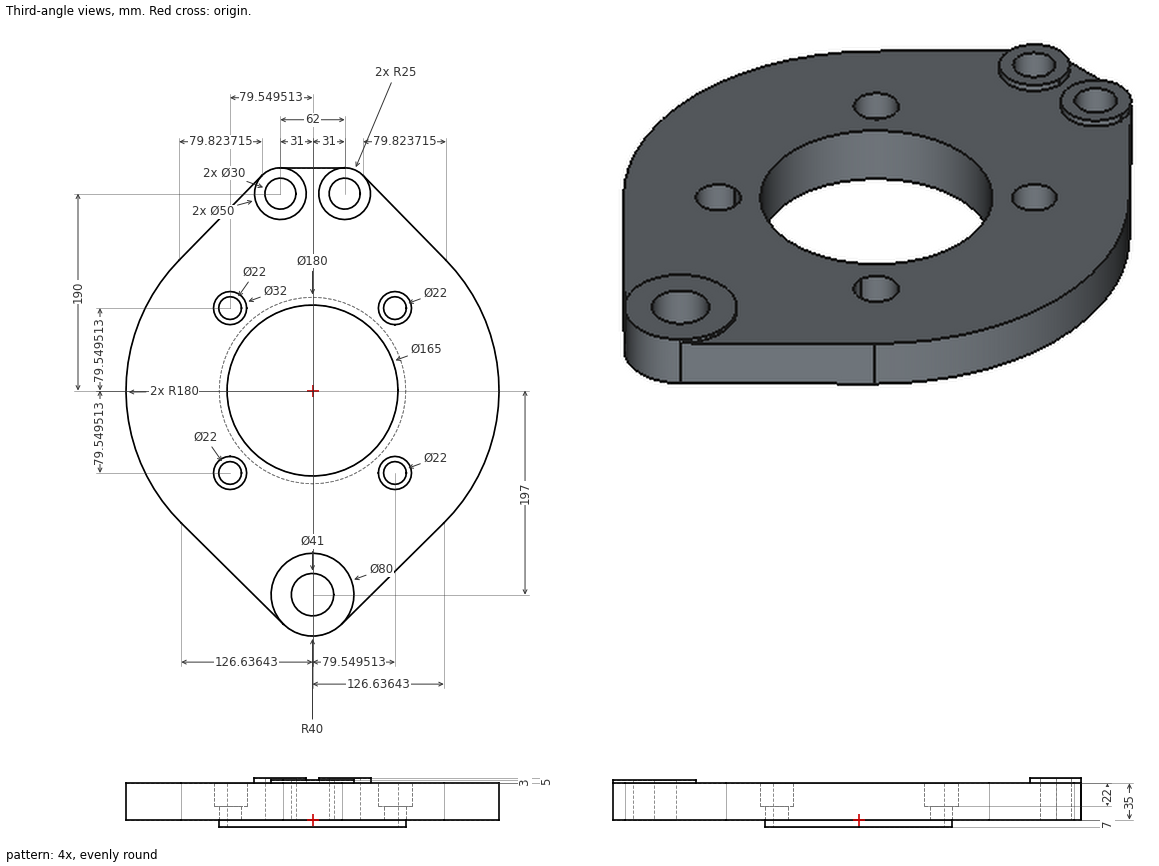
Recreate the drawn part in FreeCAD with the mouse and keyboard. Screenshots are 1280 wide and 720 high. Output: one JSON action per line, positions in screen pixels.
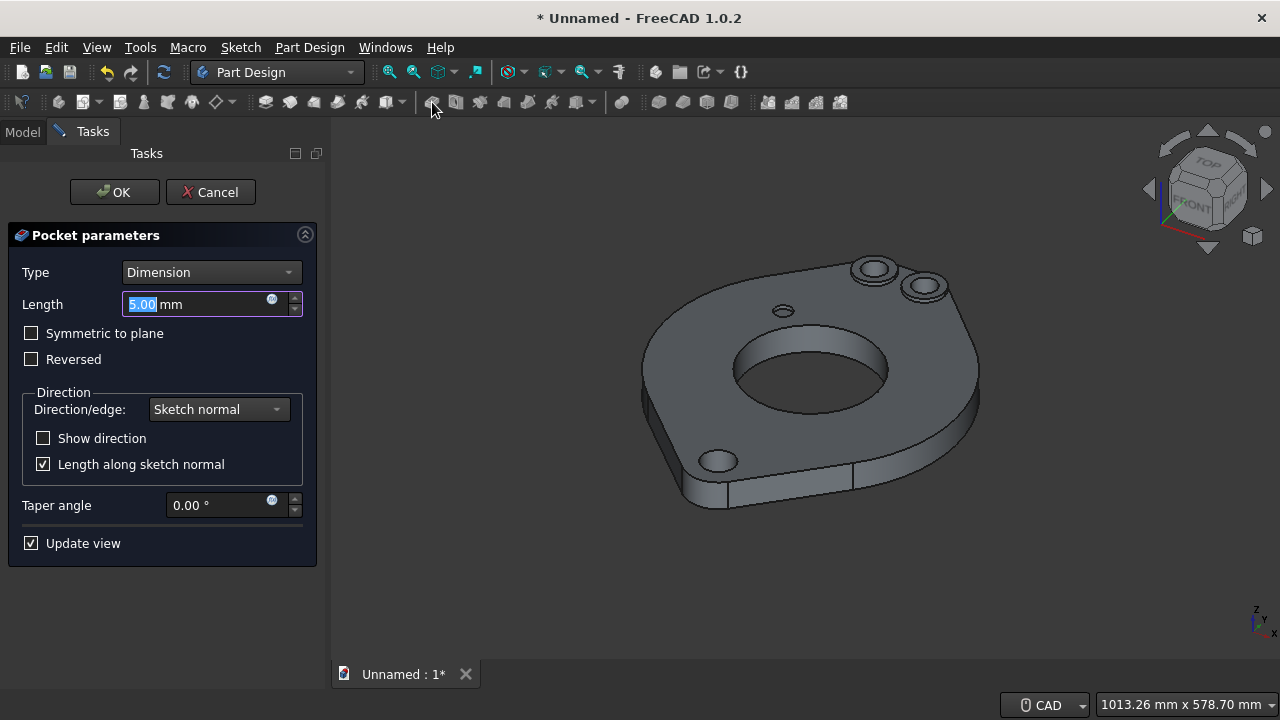
{"action": "left_click", "coordinate": [212, 272]}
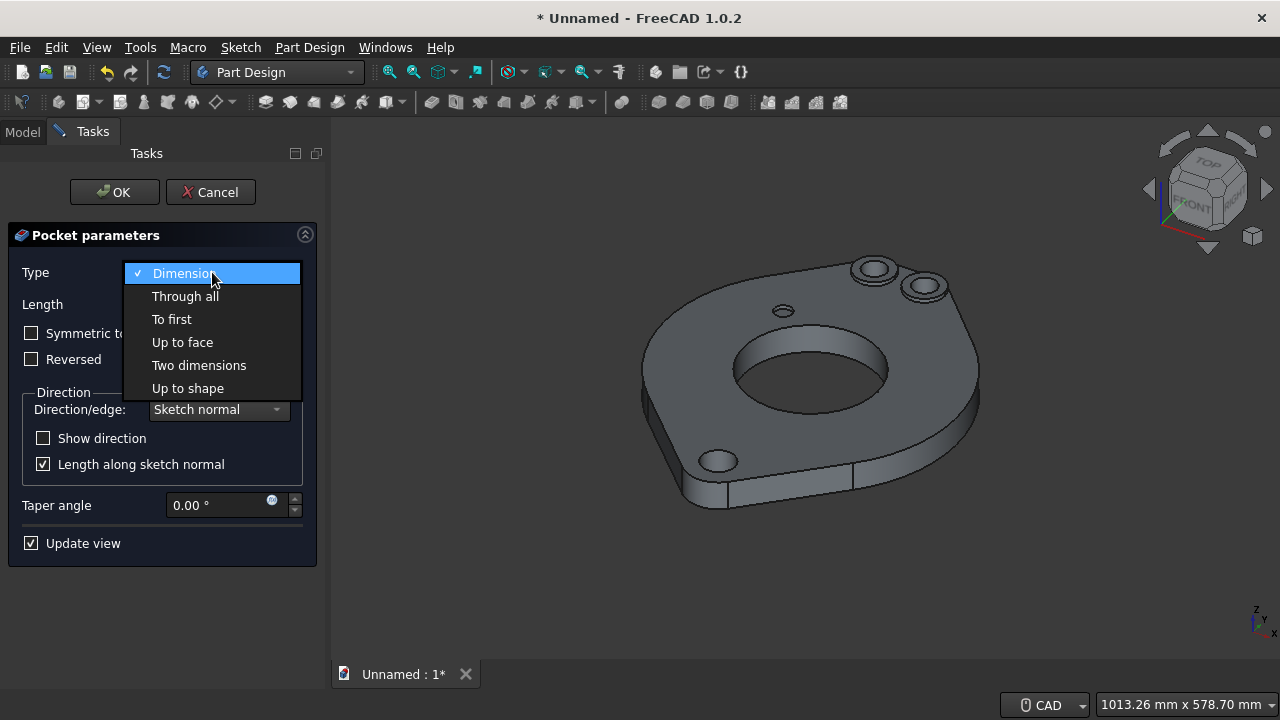
{"action": "left_click", "coordinate": [212, 320]}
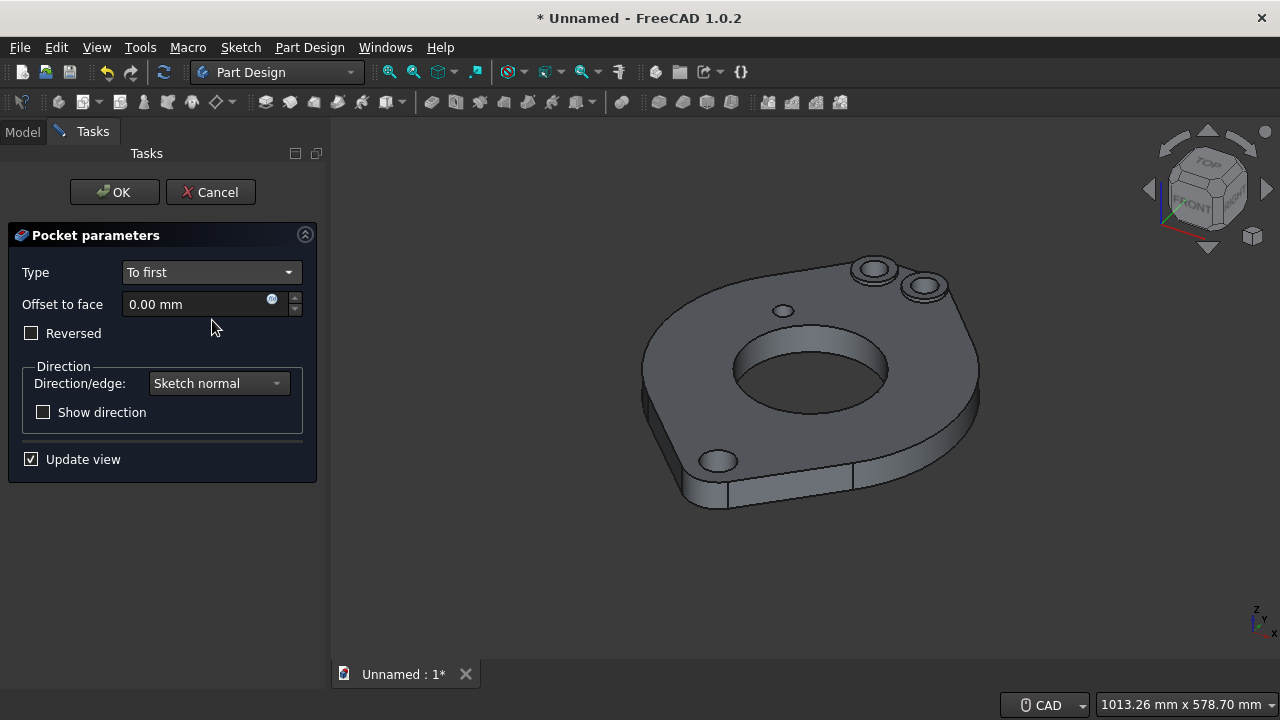
{"action": "left_click", "coordinate": [115, 192]}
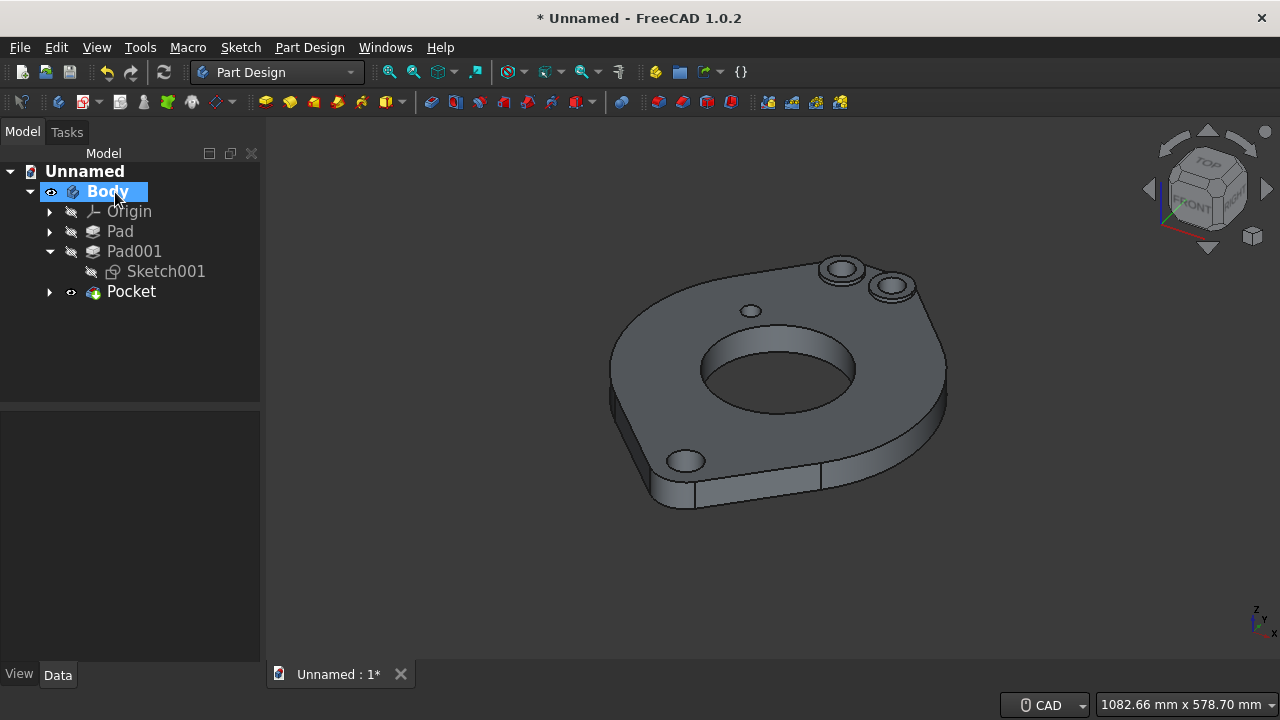
{"action": "left_click", "coordinate": [875, 327]}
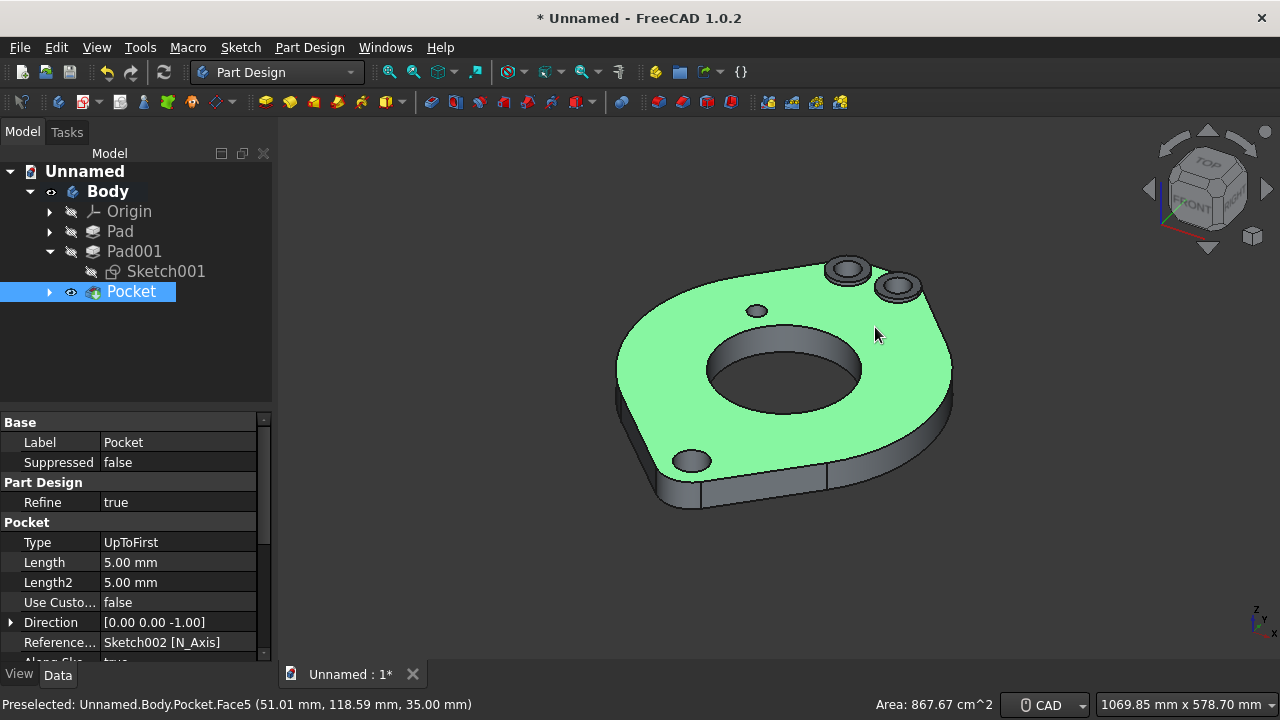
{"action": "left_click", "coordinate": [84, 102]}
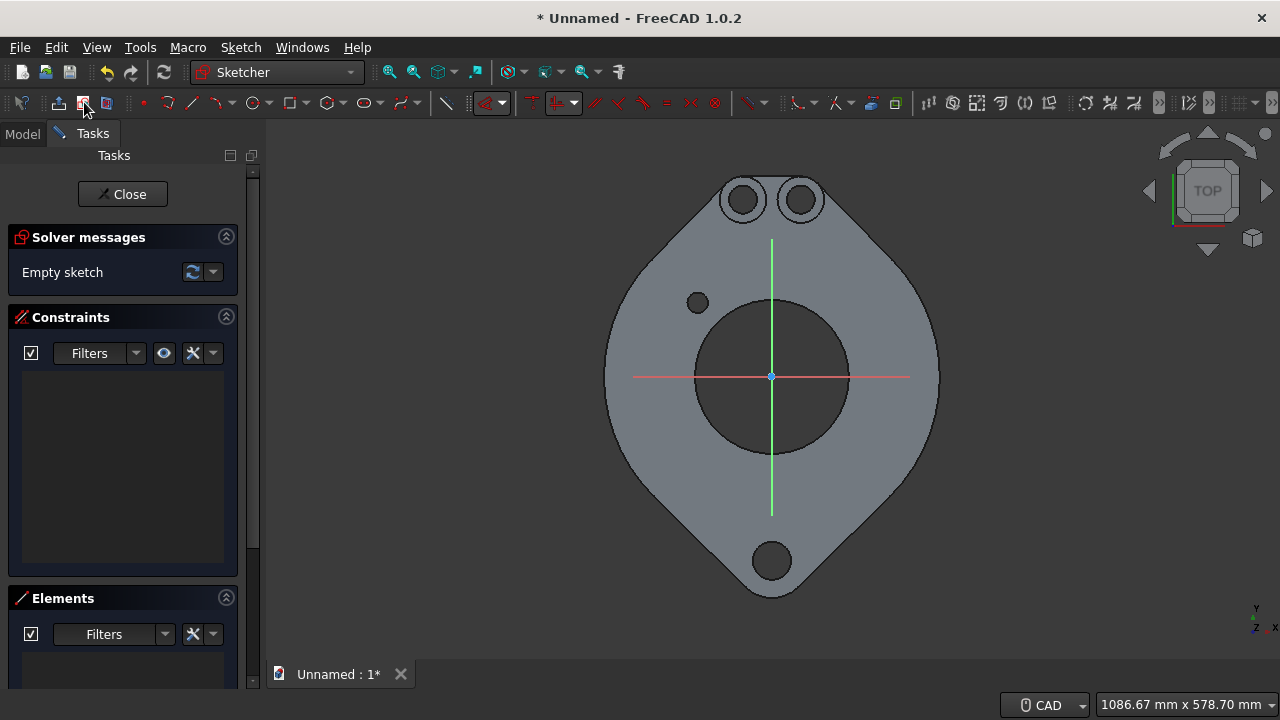
{"action": "scroll", "coordinate": [697, 455], "scroll_direction": "up", "scroll_amount": 14}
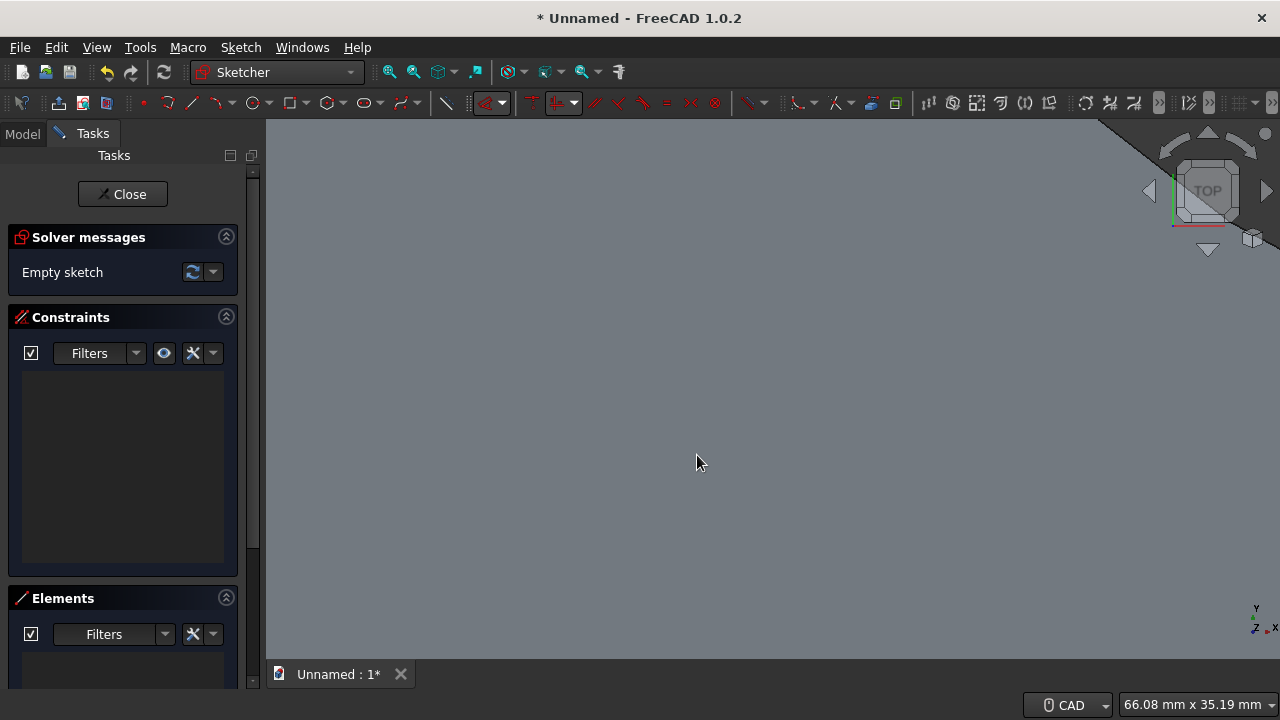
{"action": "key", "text": "g c"}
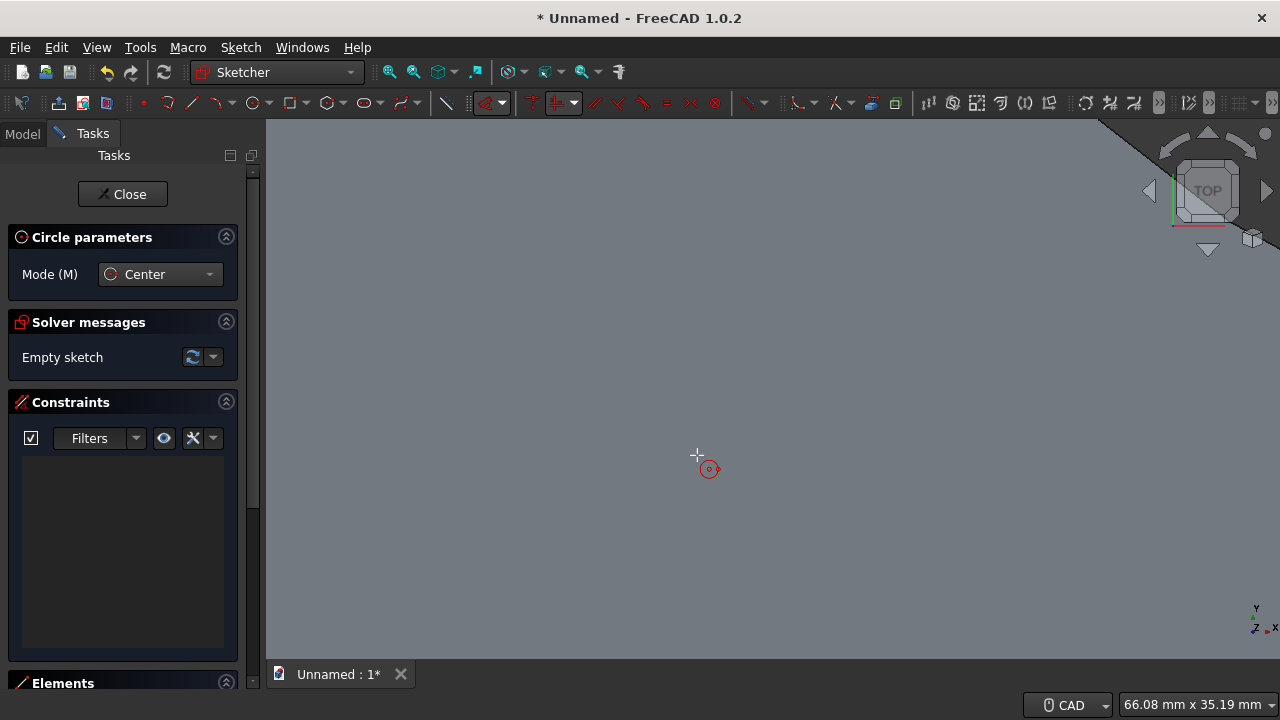
{"action": "left_click", "coordinate": [702, 383]}
{"action": "left_click", "coordinate": [821, 263]}
{"action": "key", "text": "Escape"}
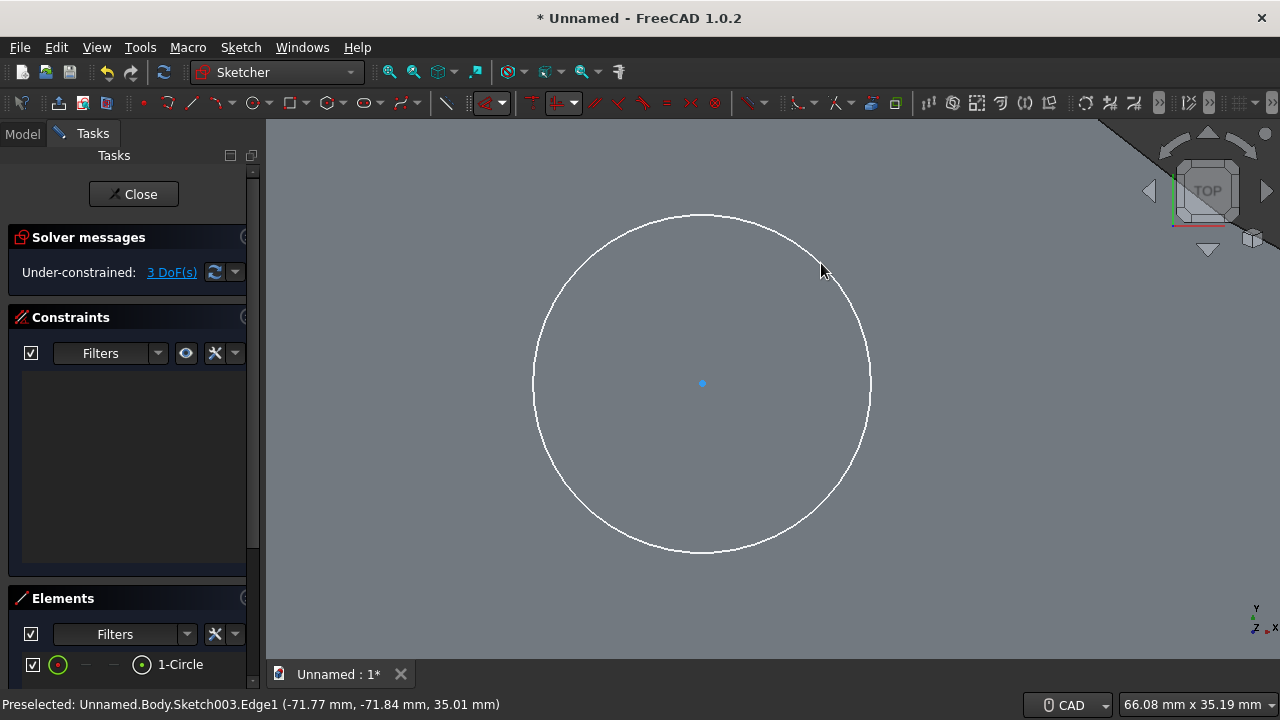
{"action": "left_click", "coordinate": [821, 264]}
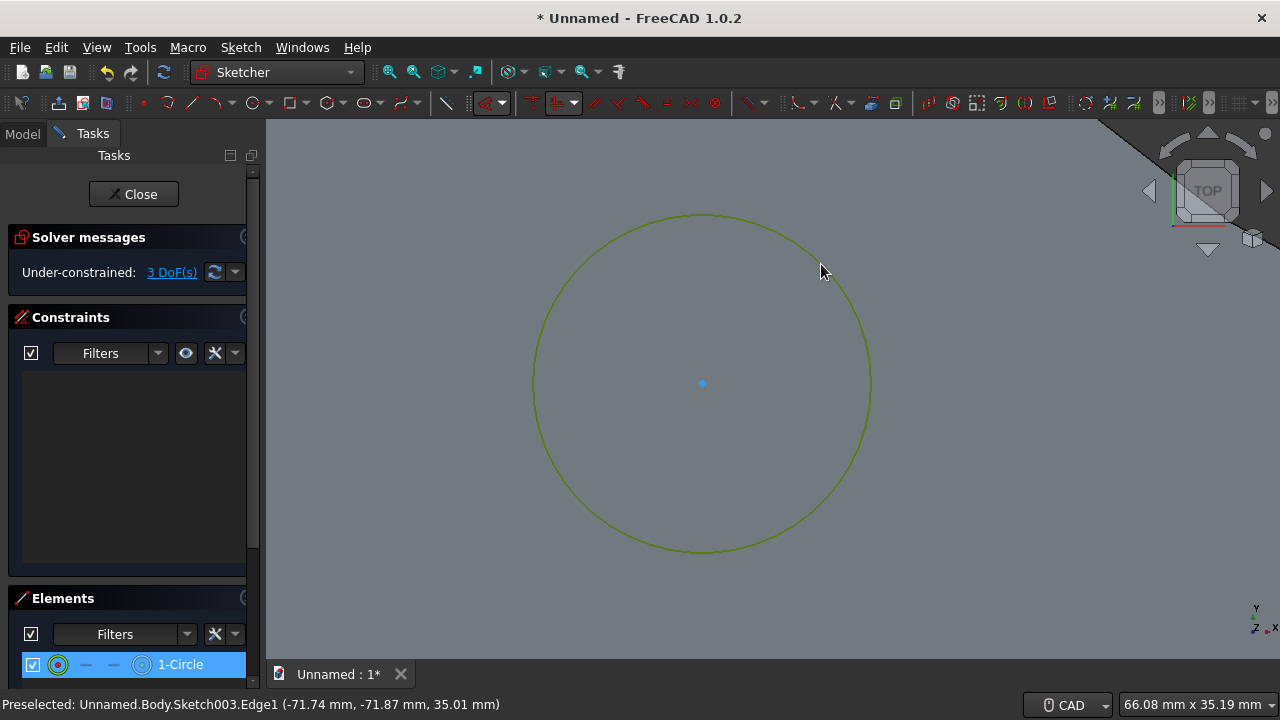
{"action": "left_click", "coordinate": [504, 104]}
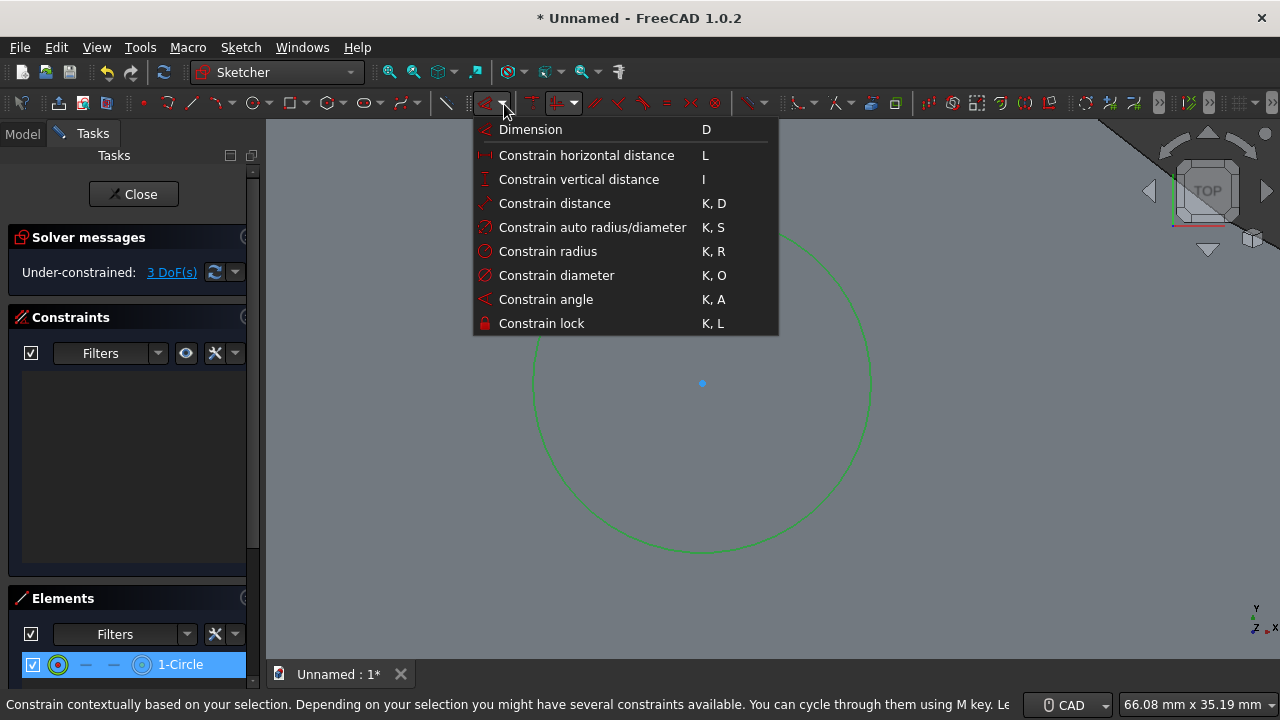
{"action": "left_click", "coordinate": [626, 275]}